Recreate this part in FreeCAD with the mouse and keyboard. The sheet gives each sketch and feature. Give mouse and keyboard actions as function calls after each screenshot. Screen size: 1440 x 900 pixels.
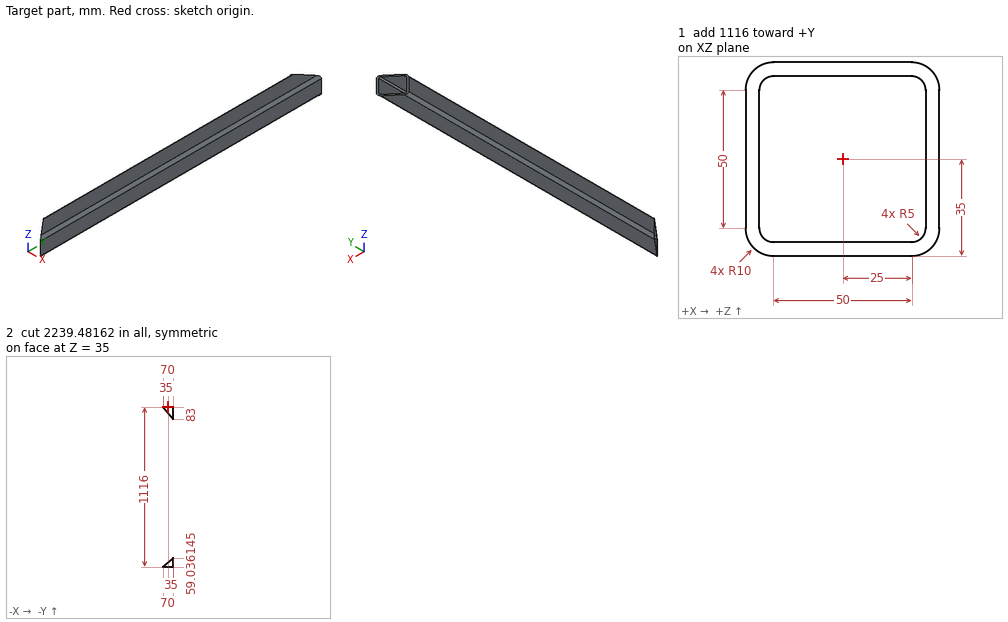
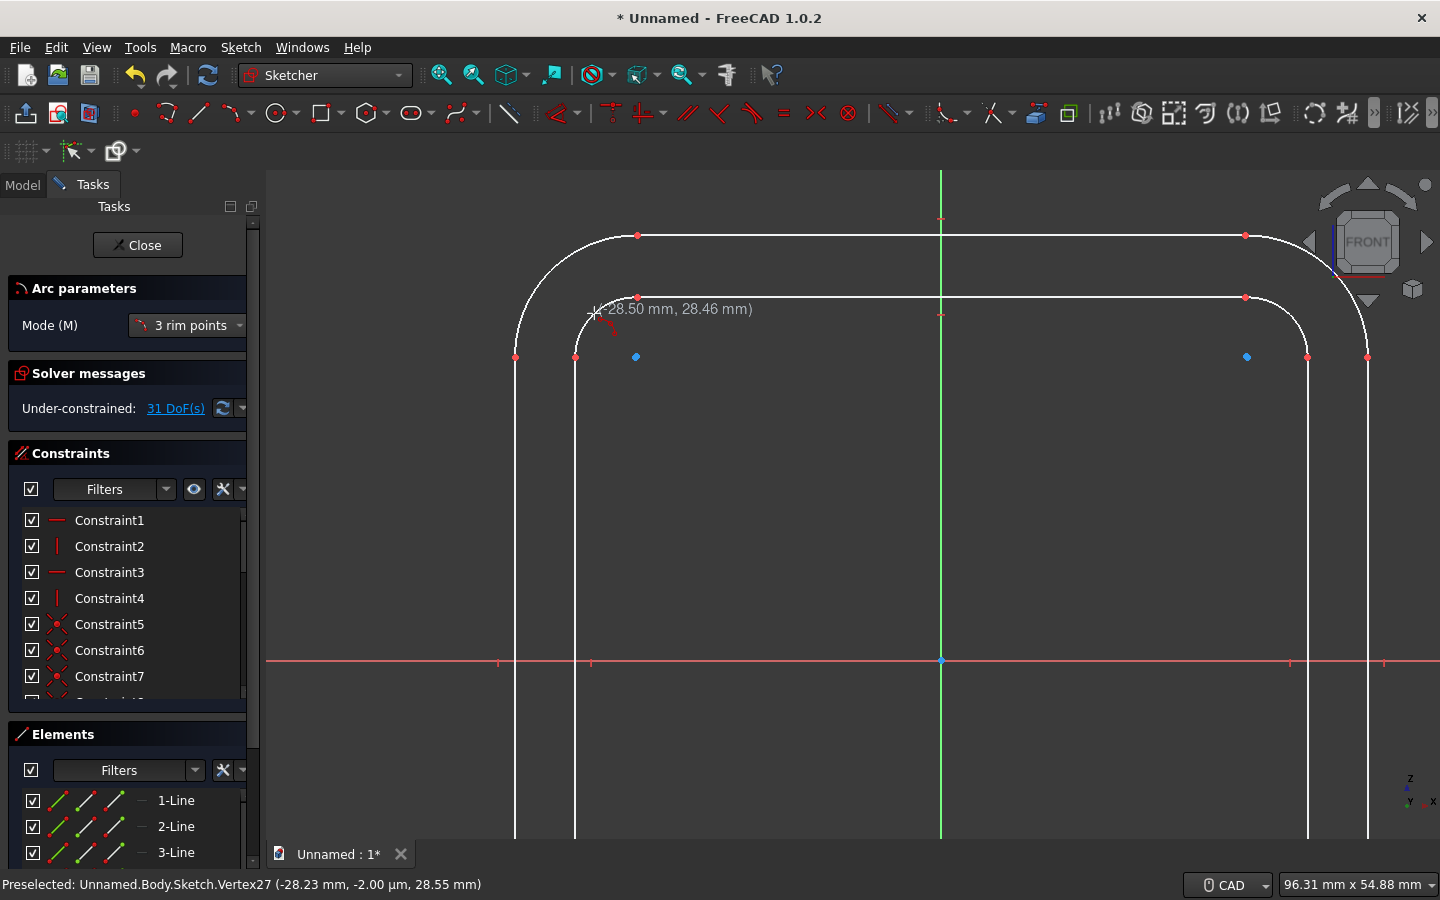
scroll(594, 314, down, 3)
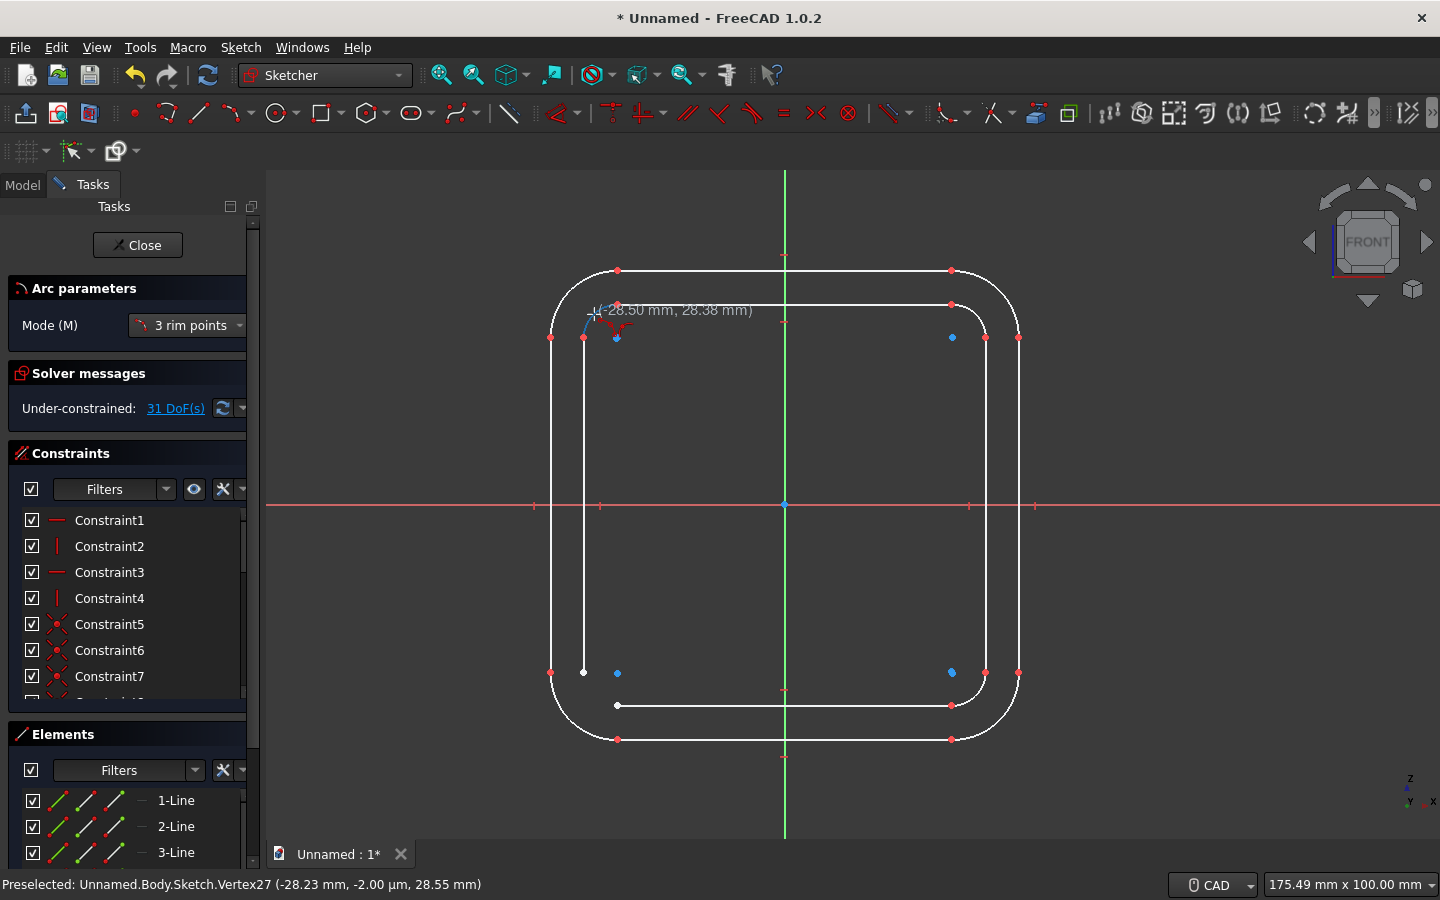
click(584, 673)
click(618, 706)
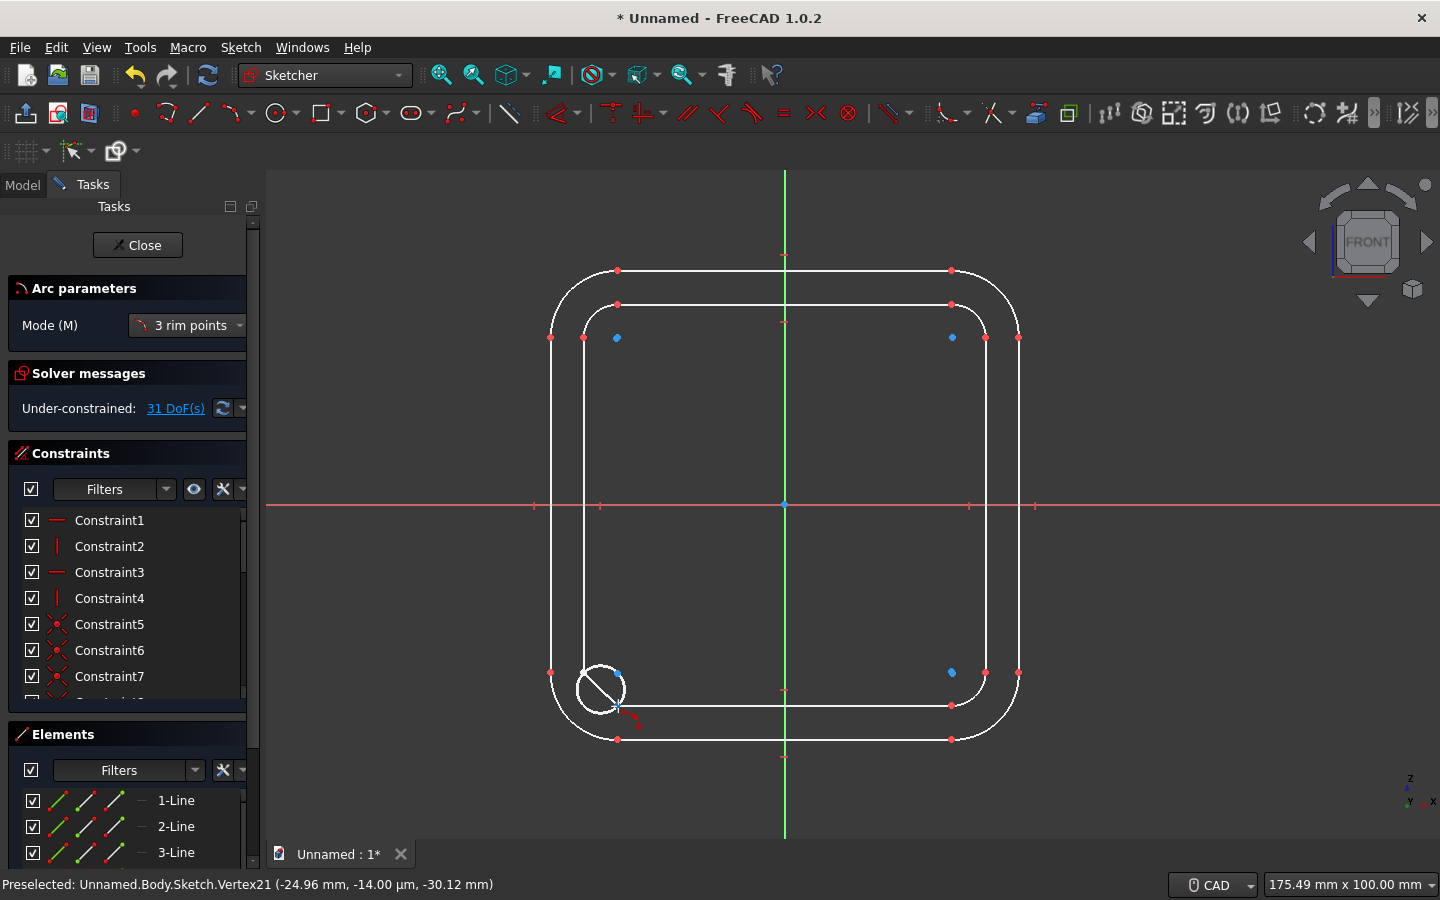
scroll(594, 695, up, 3)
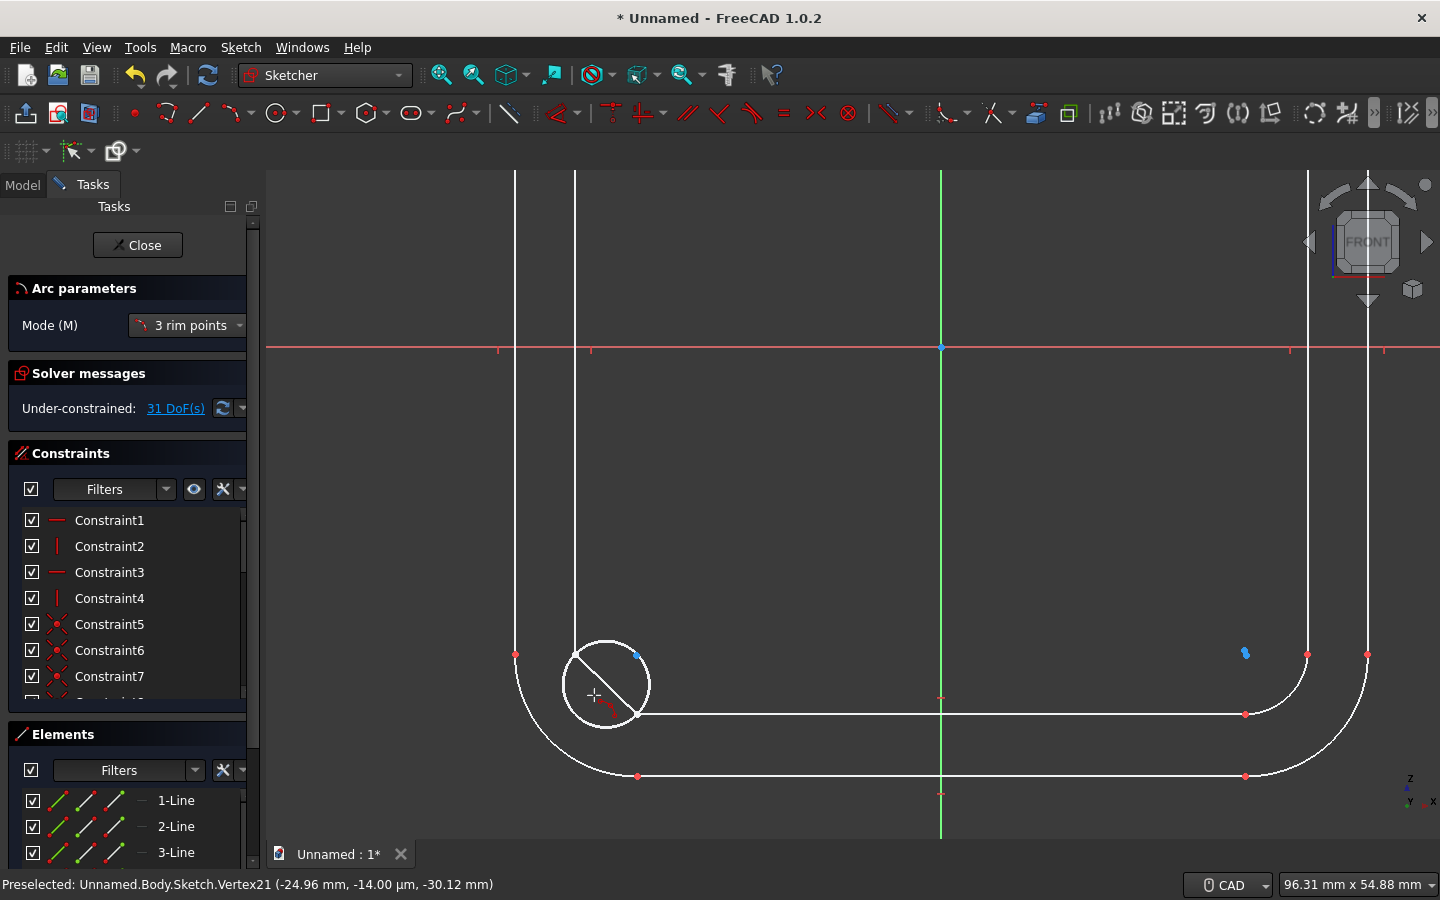
click(594, 695)
key(Escape)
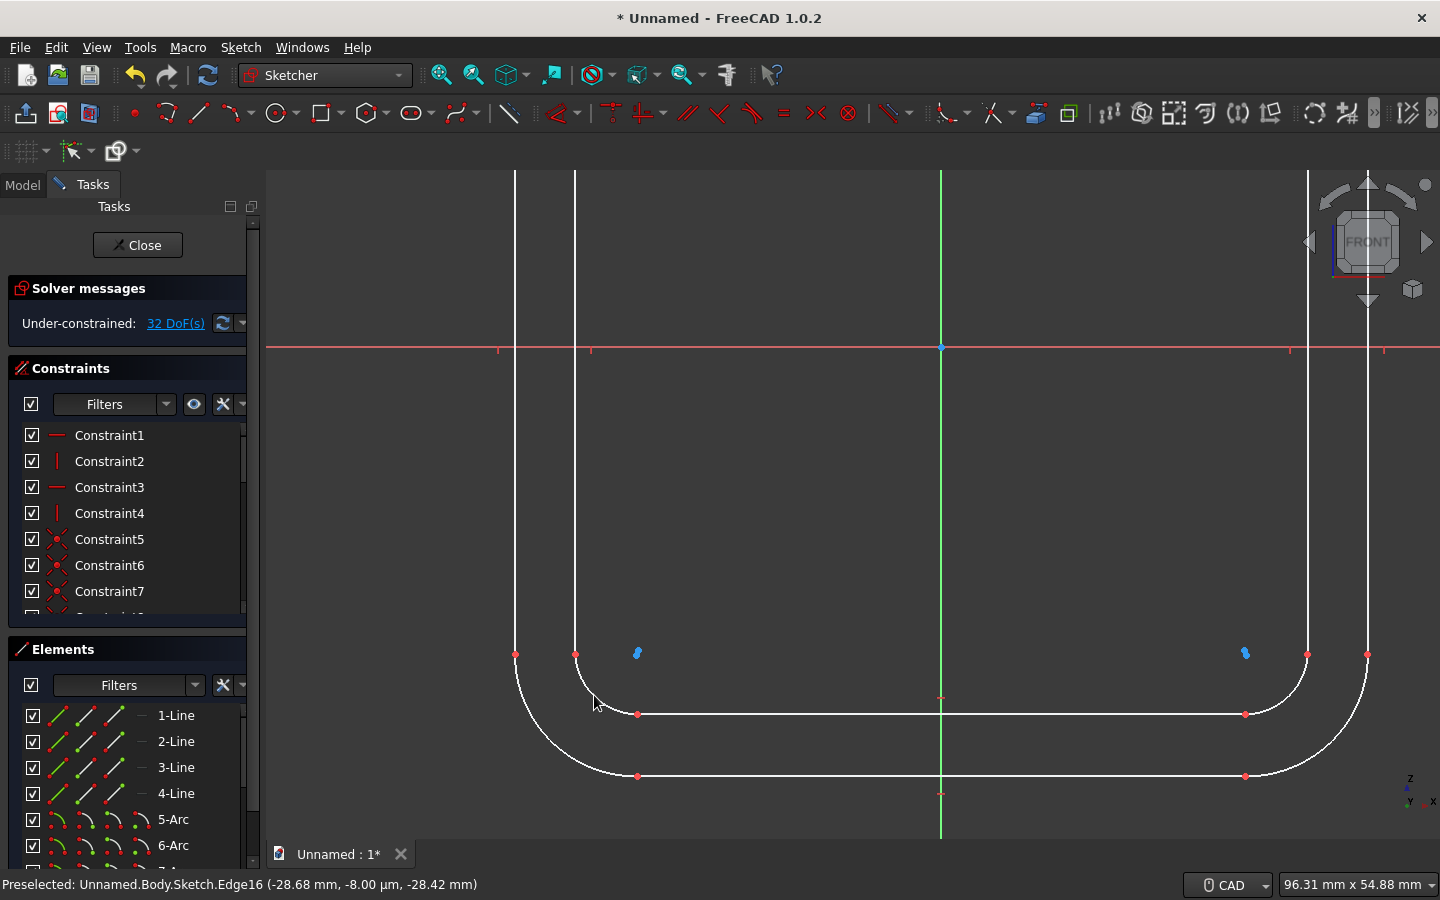
click(1063, 776)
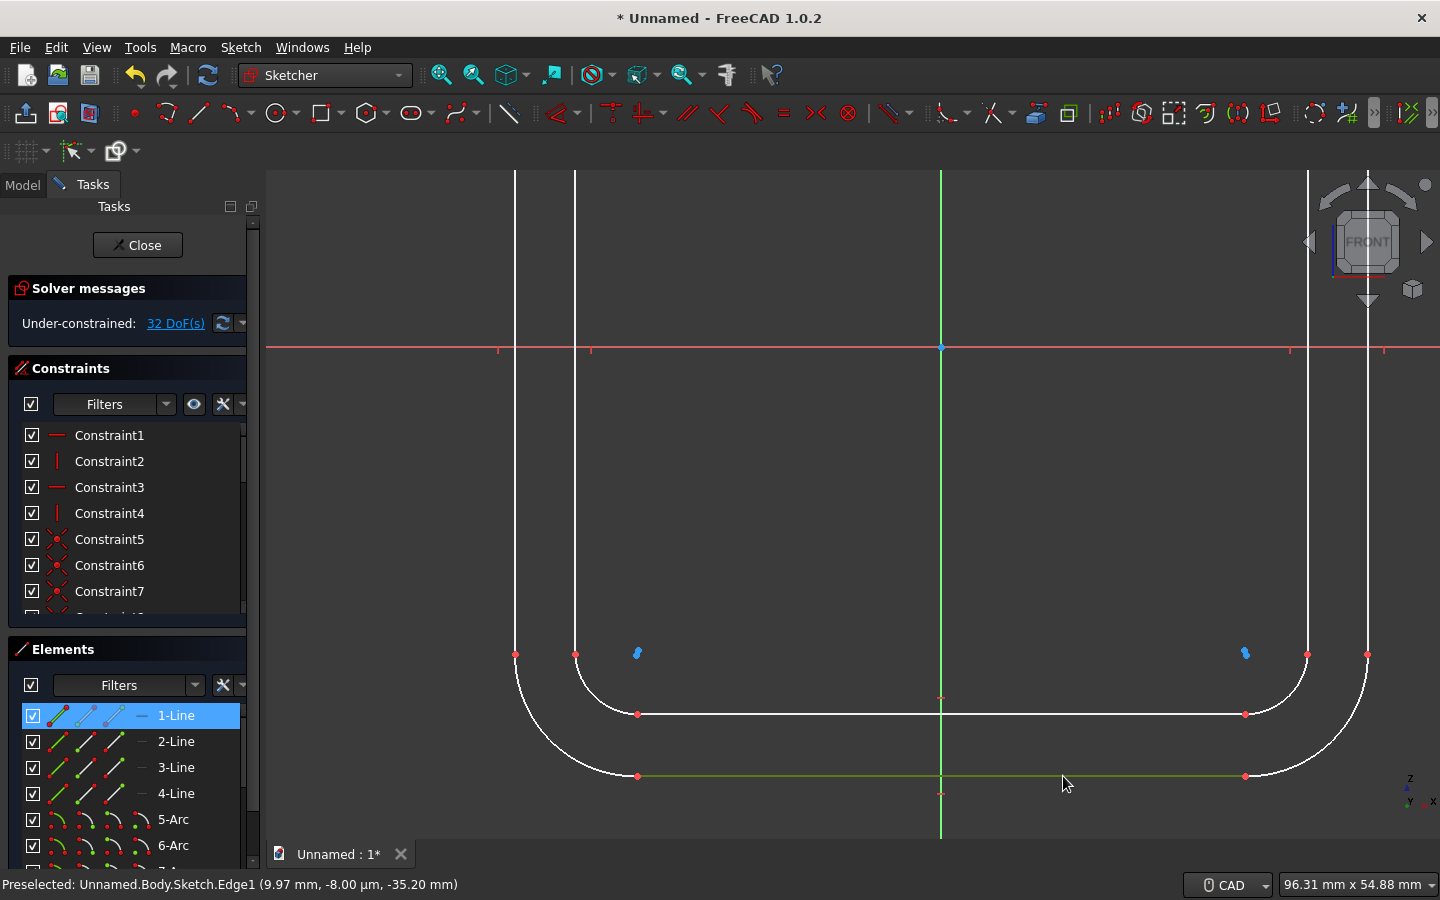
click(528, 710)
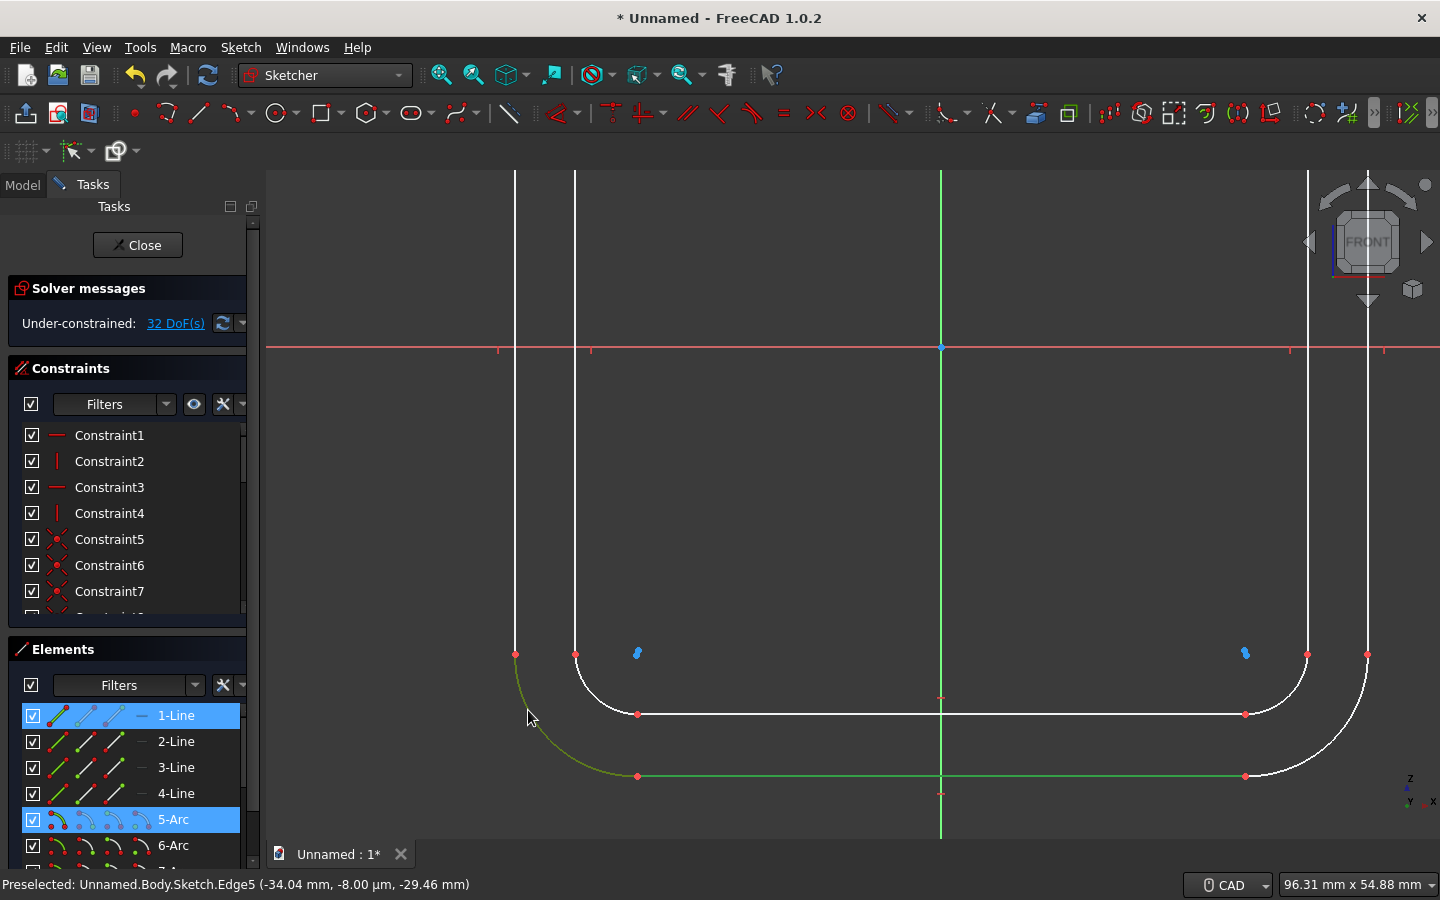
key(t)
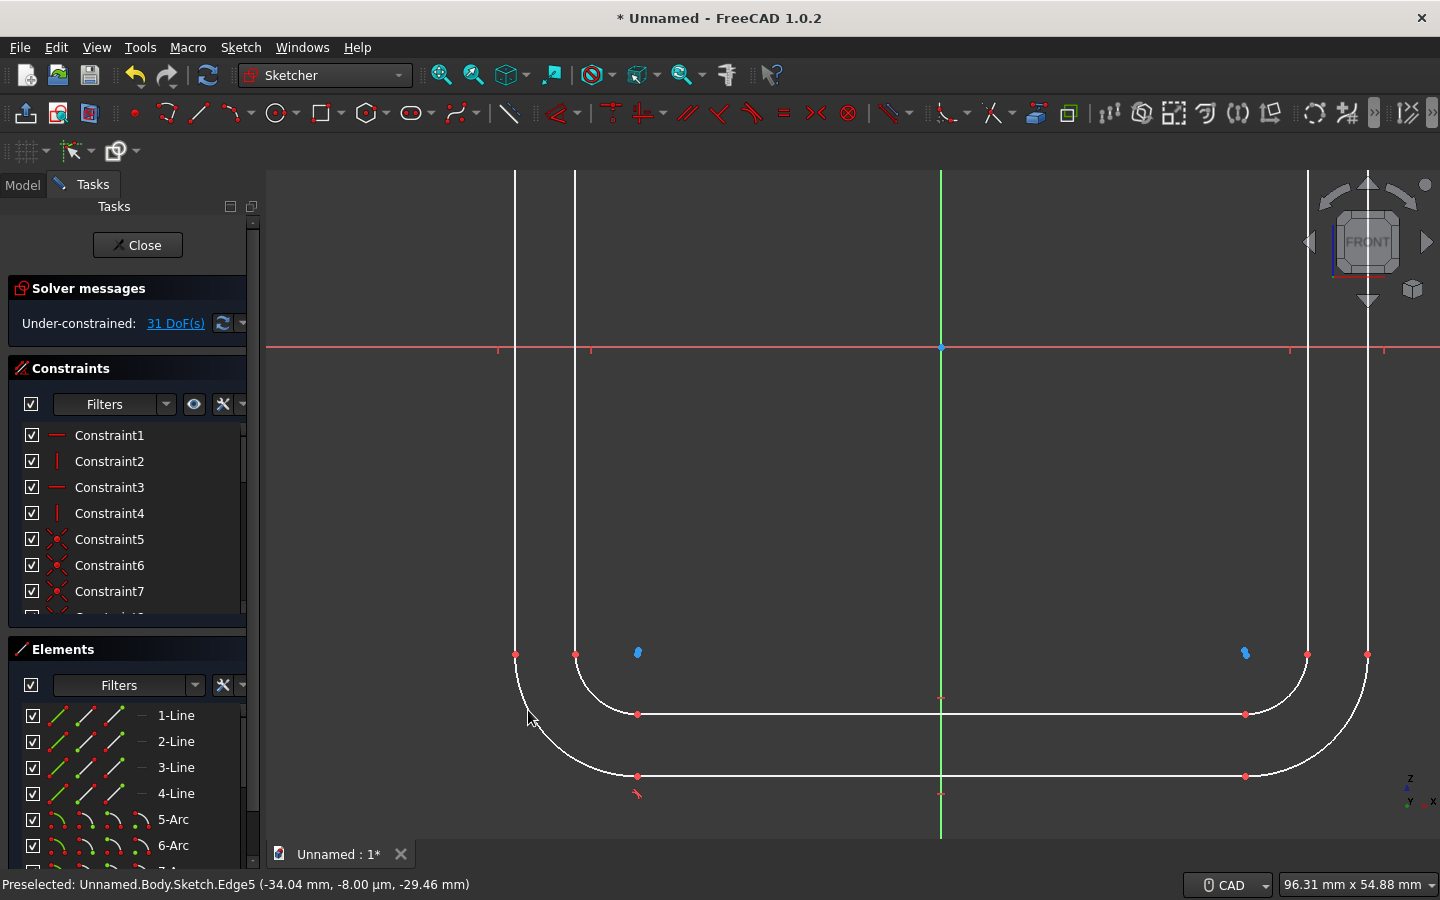
click(1063, 776)